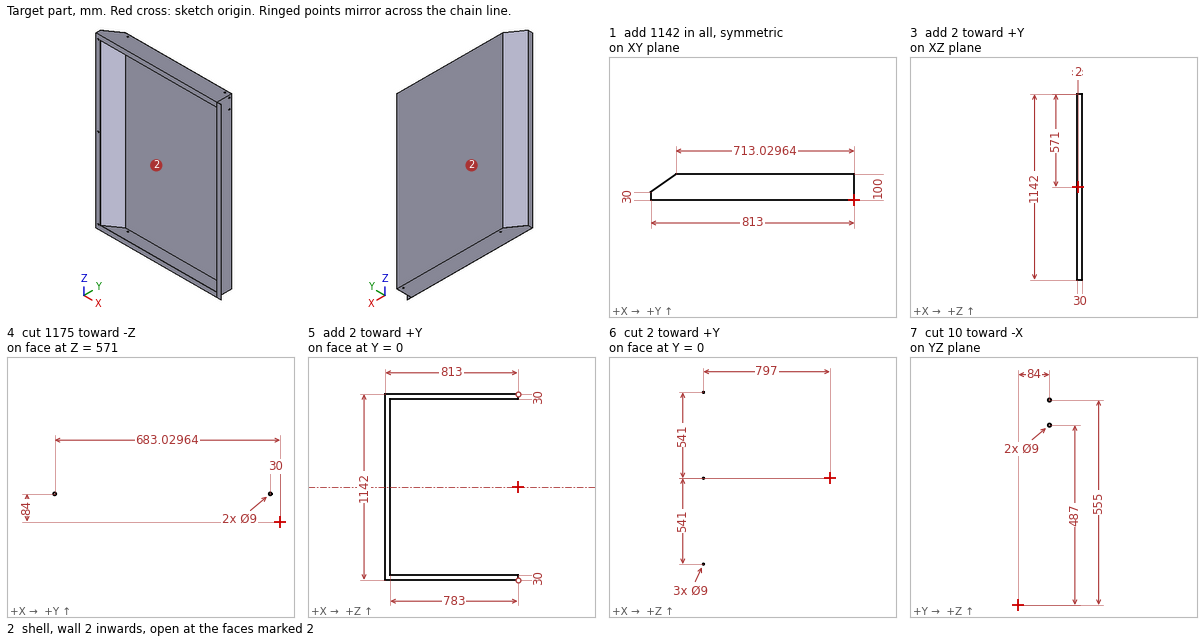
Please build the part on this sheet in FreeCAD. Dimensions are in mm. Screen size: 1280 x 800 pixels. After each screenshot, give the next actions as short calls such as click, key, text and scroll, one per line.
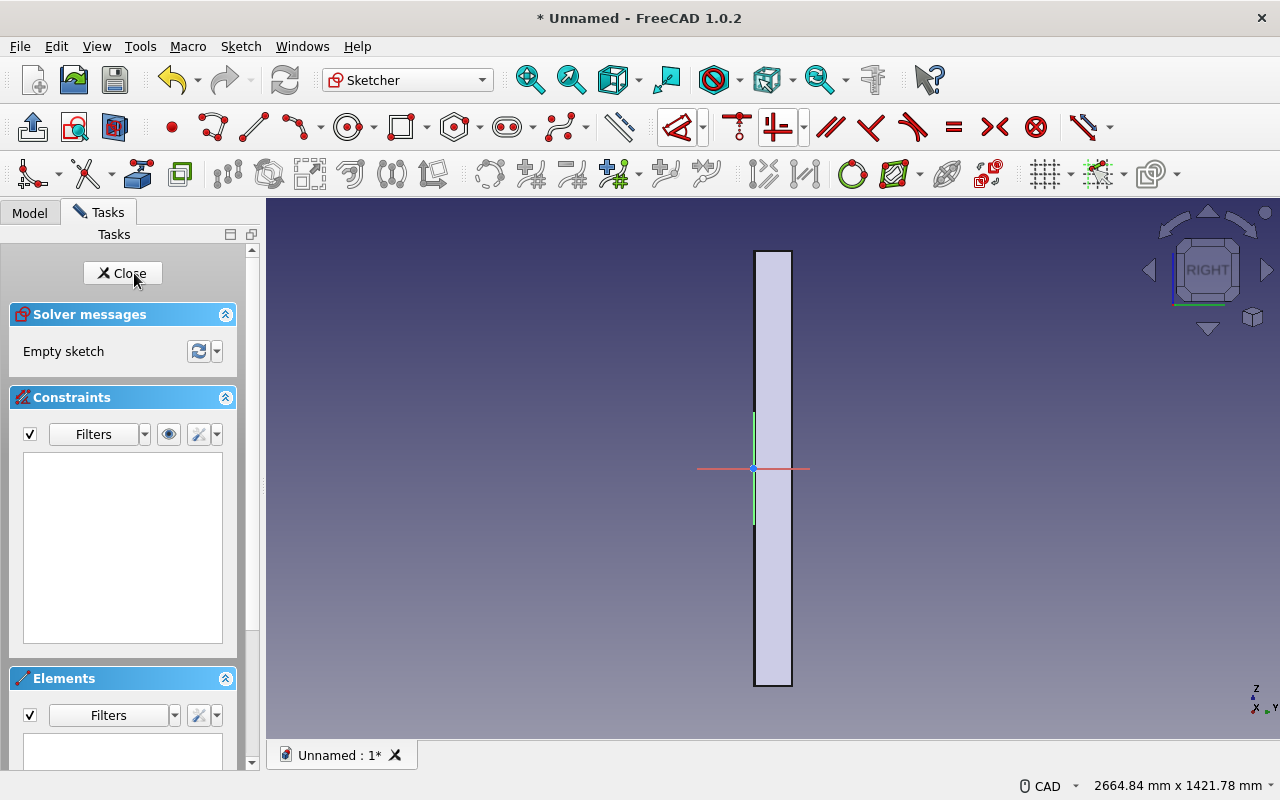
scroll(794, 250, up, 12)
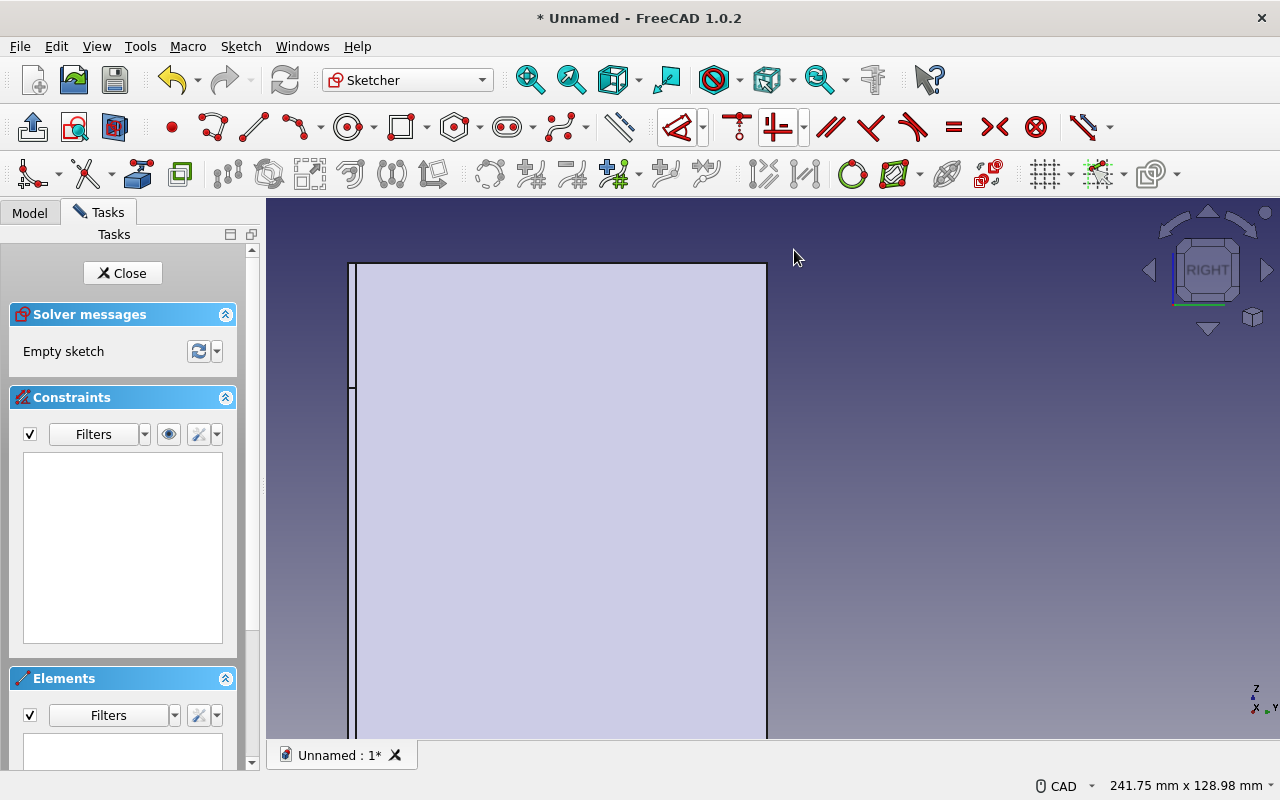
click(348, 128)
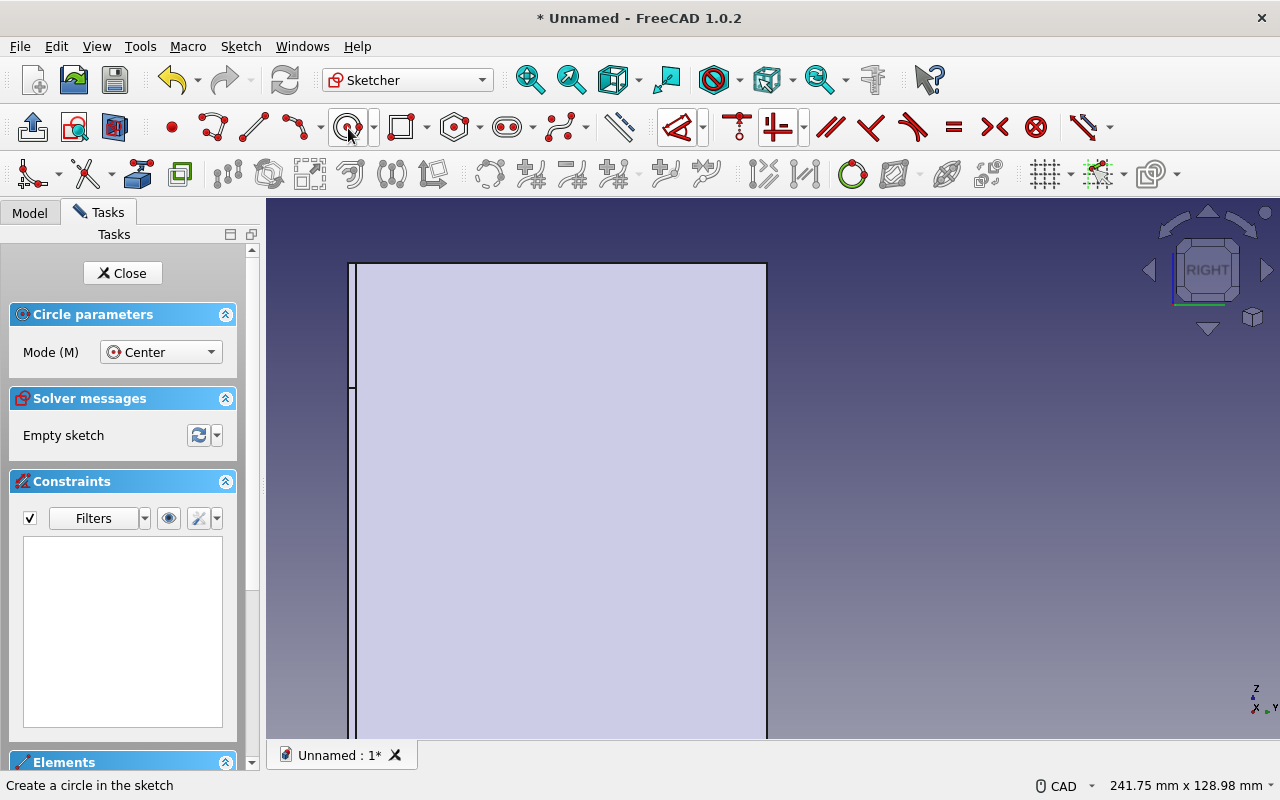
click(700, 330)
click(713, 316)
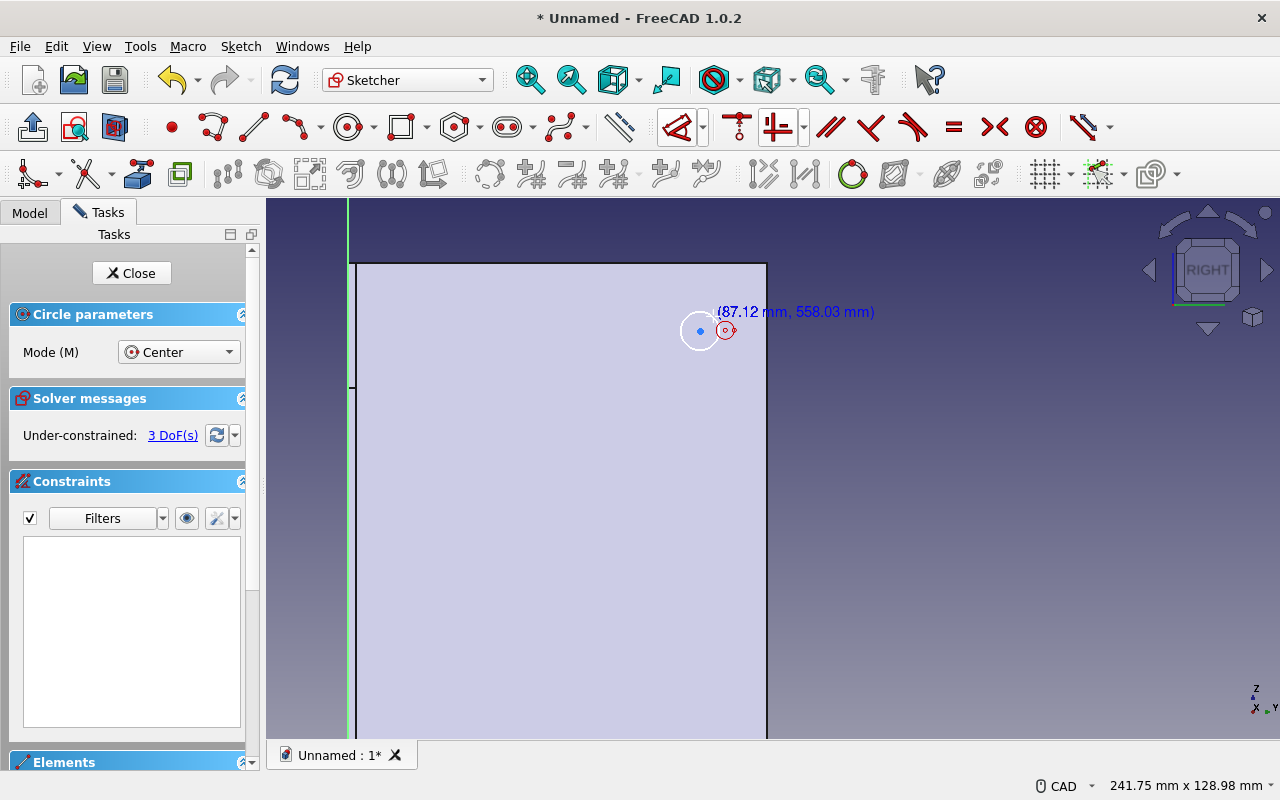
click(700, 615)
click(713, 602)
key(Escape)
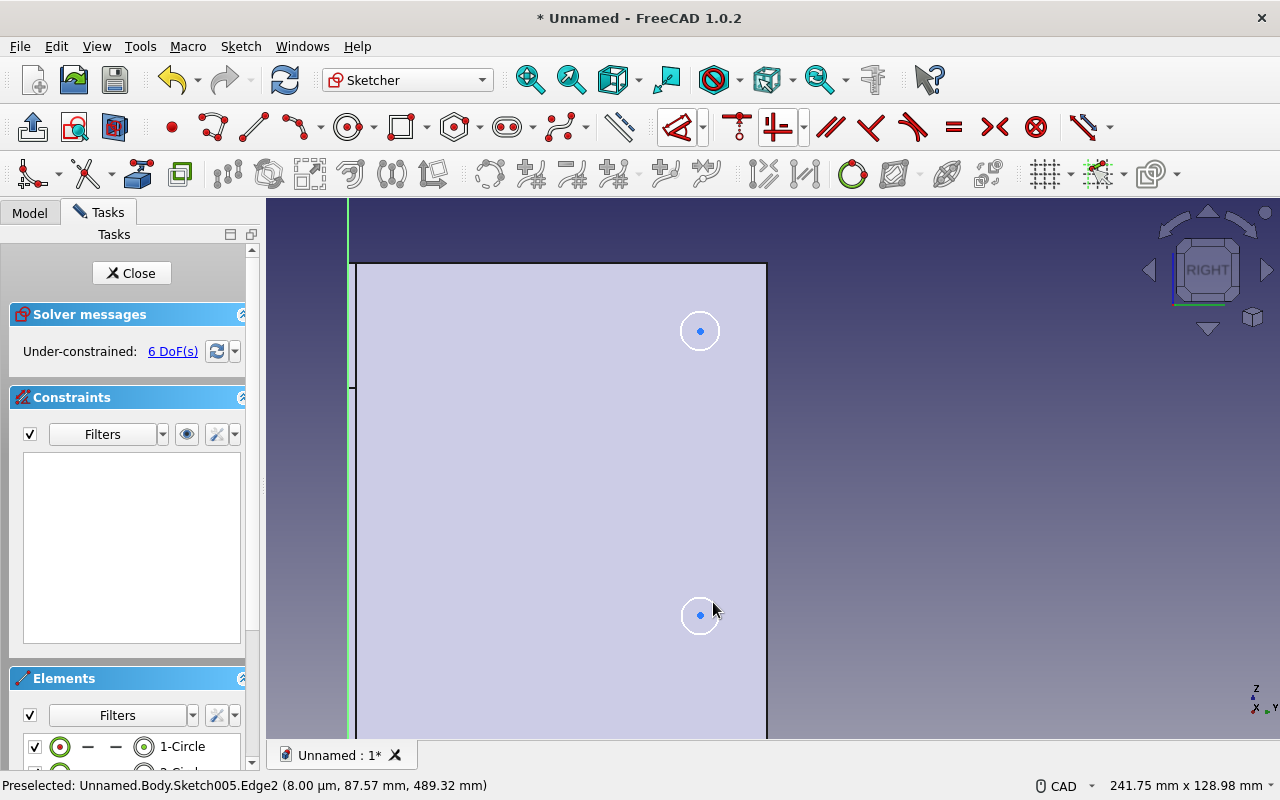
click(713, 317)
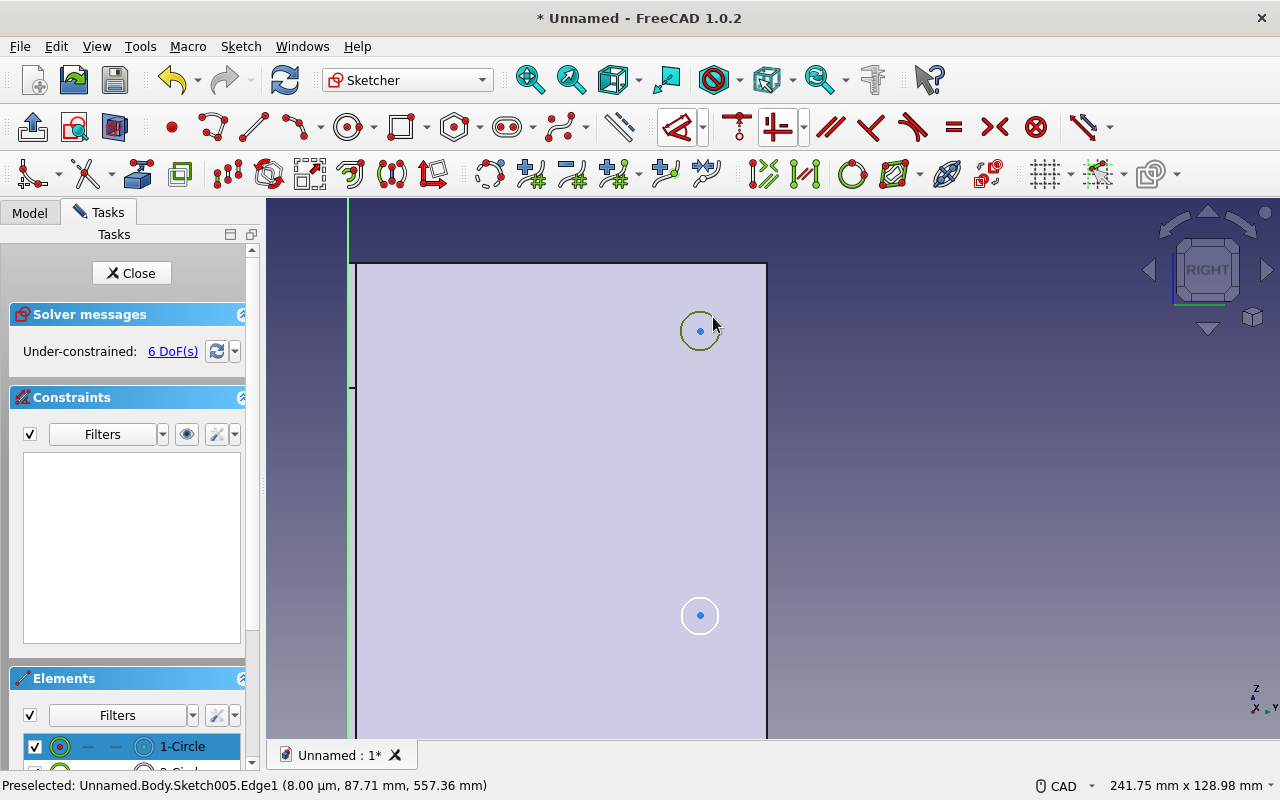
click(713, 603)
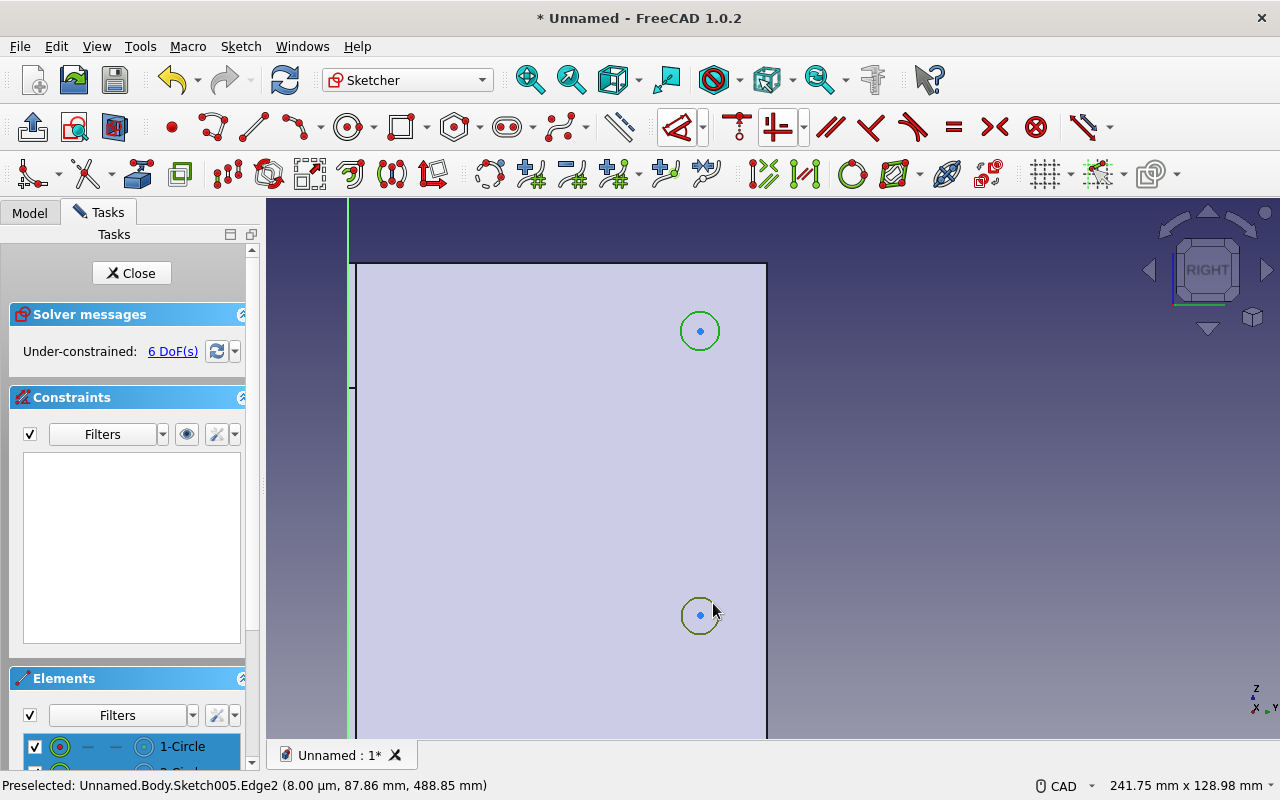
click(954, 128)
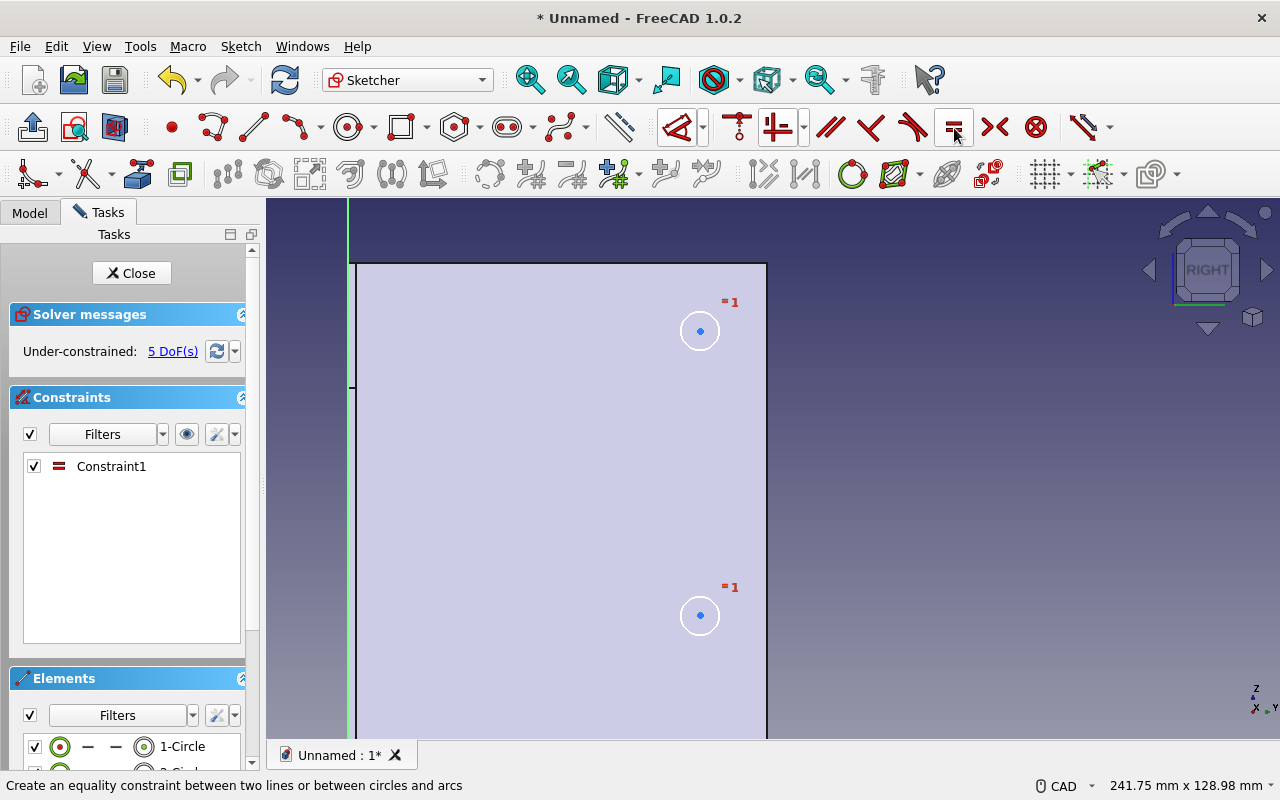
click(700, 331)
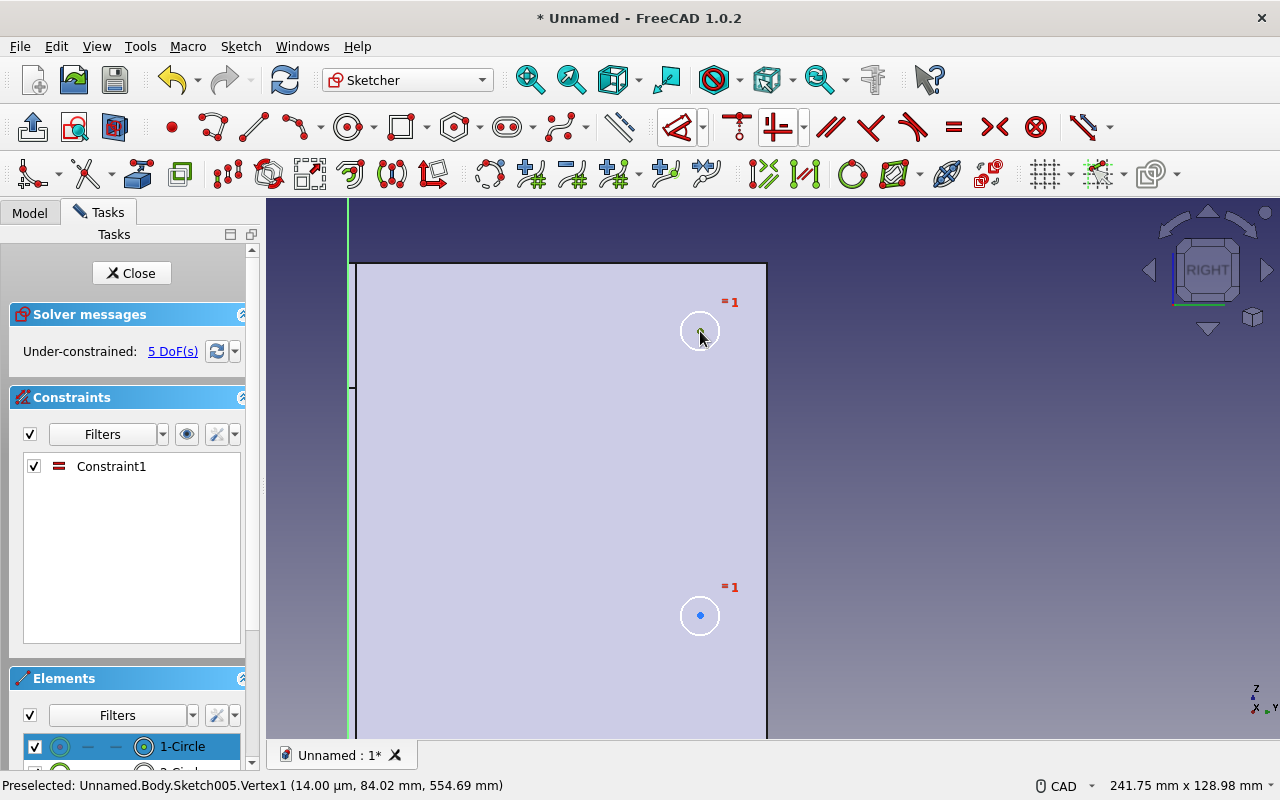
click(700, 616)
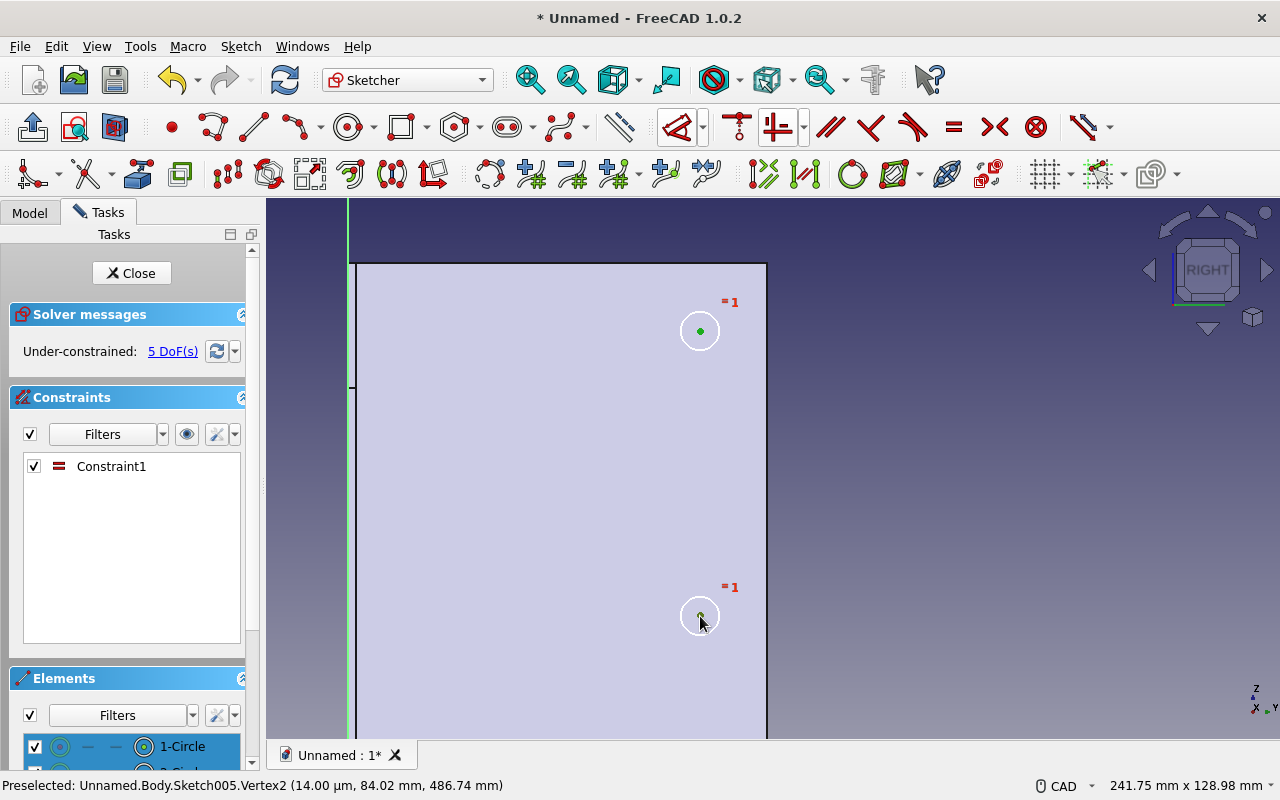
key(v)